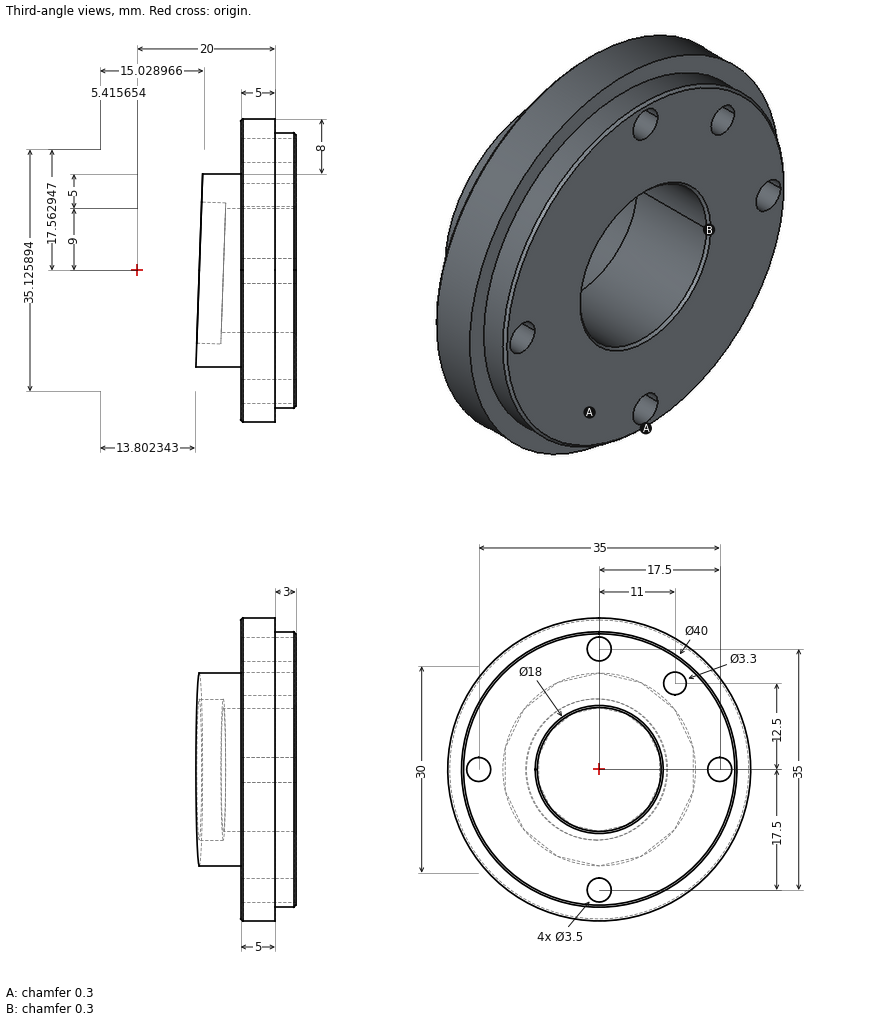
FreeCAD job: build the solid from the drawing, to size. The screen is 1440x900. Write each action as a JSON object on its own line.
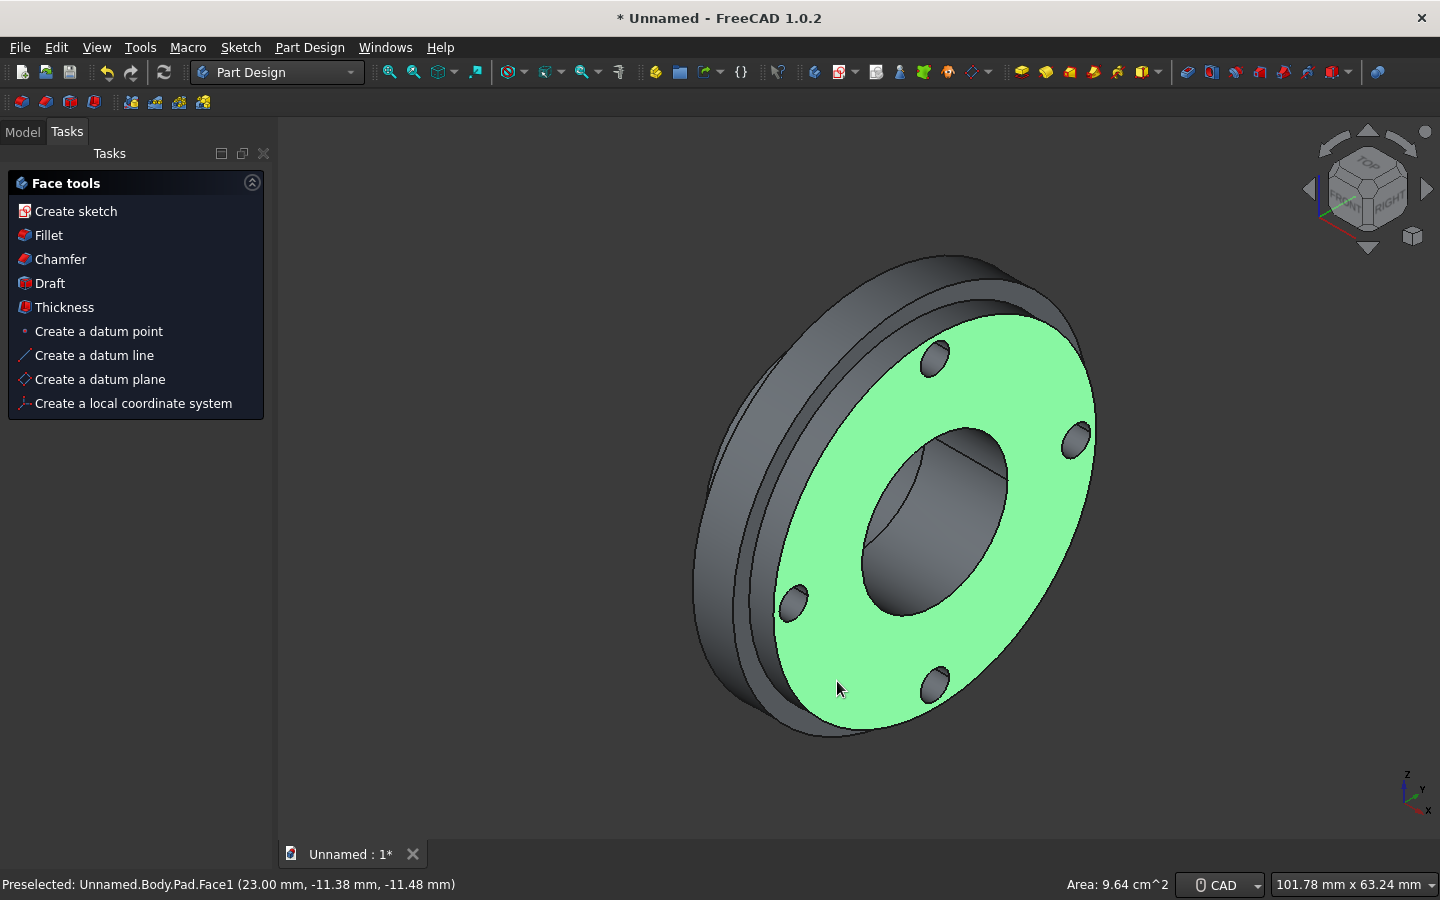
{"action": "left_click", "coordinate": [840, 72]}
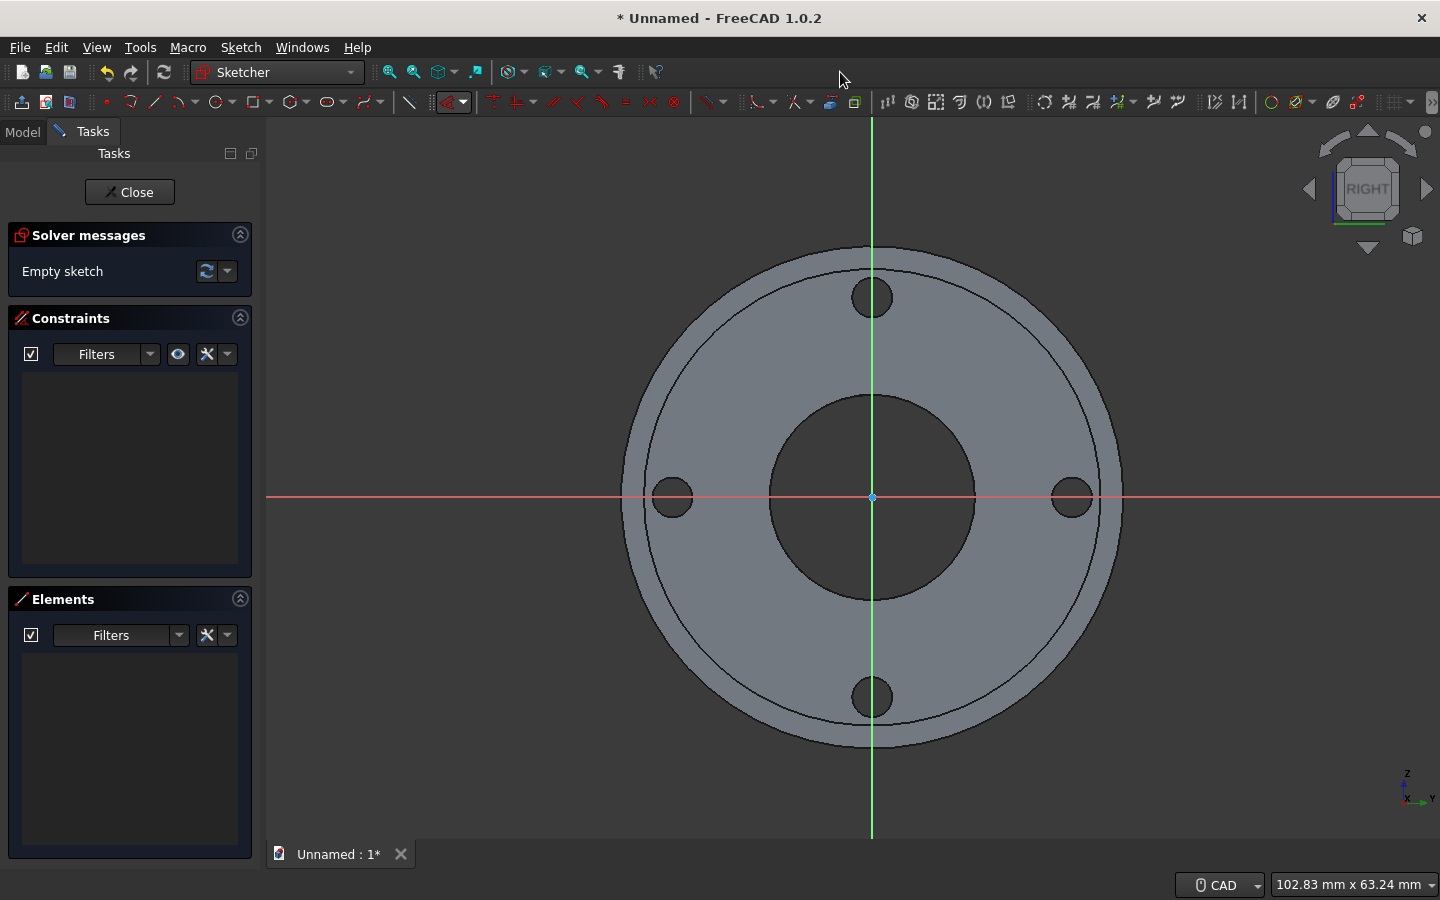
{"action": "scroll", "coordinate": [1015, 345], "scroll_direction": "up", "scroll_amount": 13}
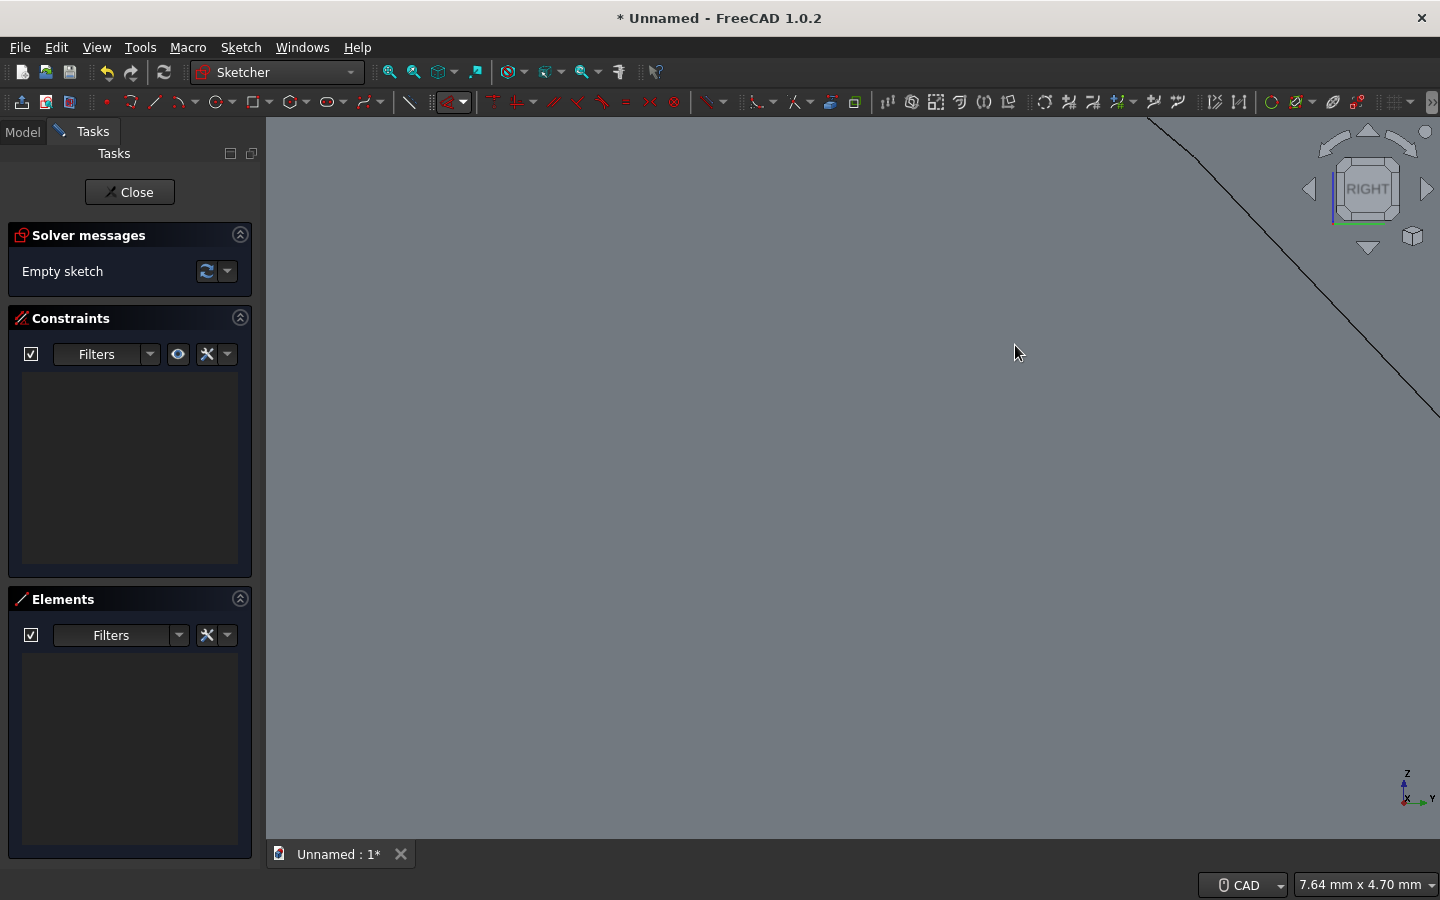
{"action": "key", "text": "g c"}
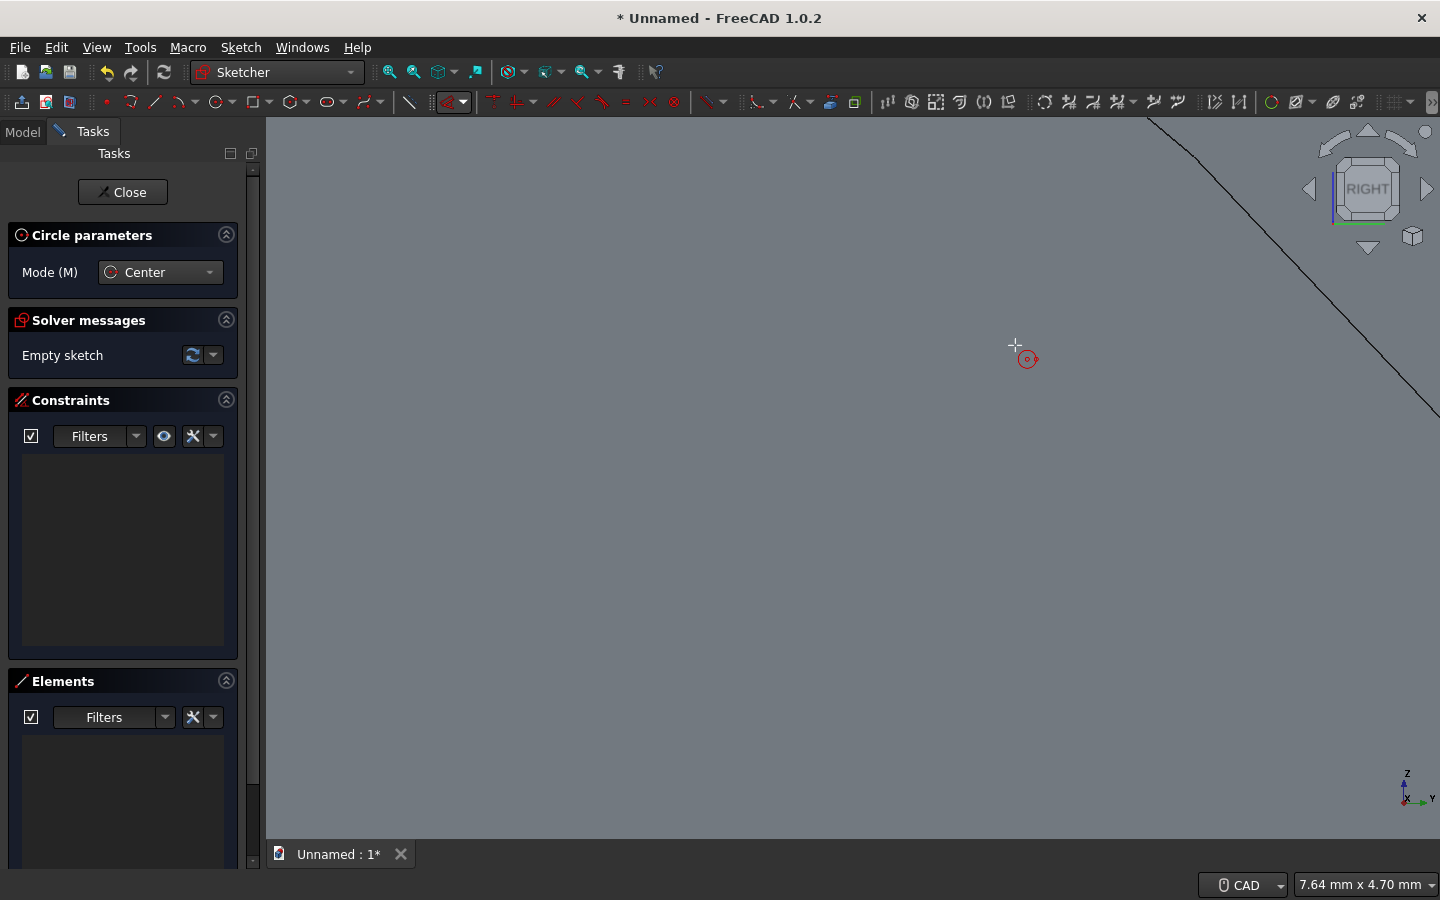
{"action": "left_click", "coordinate": [775, 472]}
{"action": "mouse_move", "coordinate": [955, 292]}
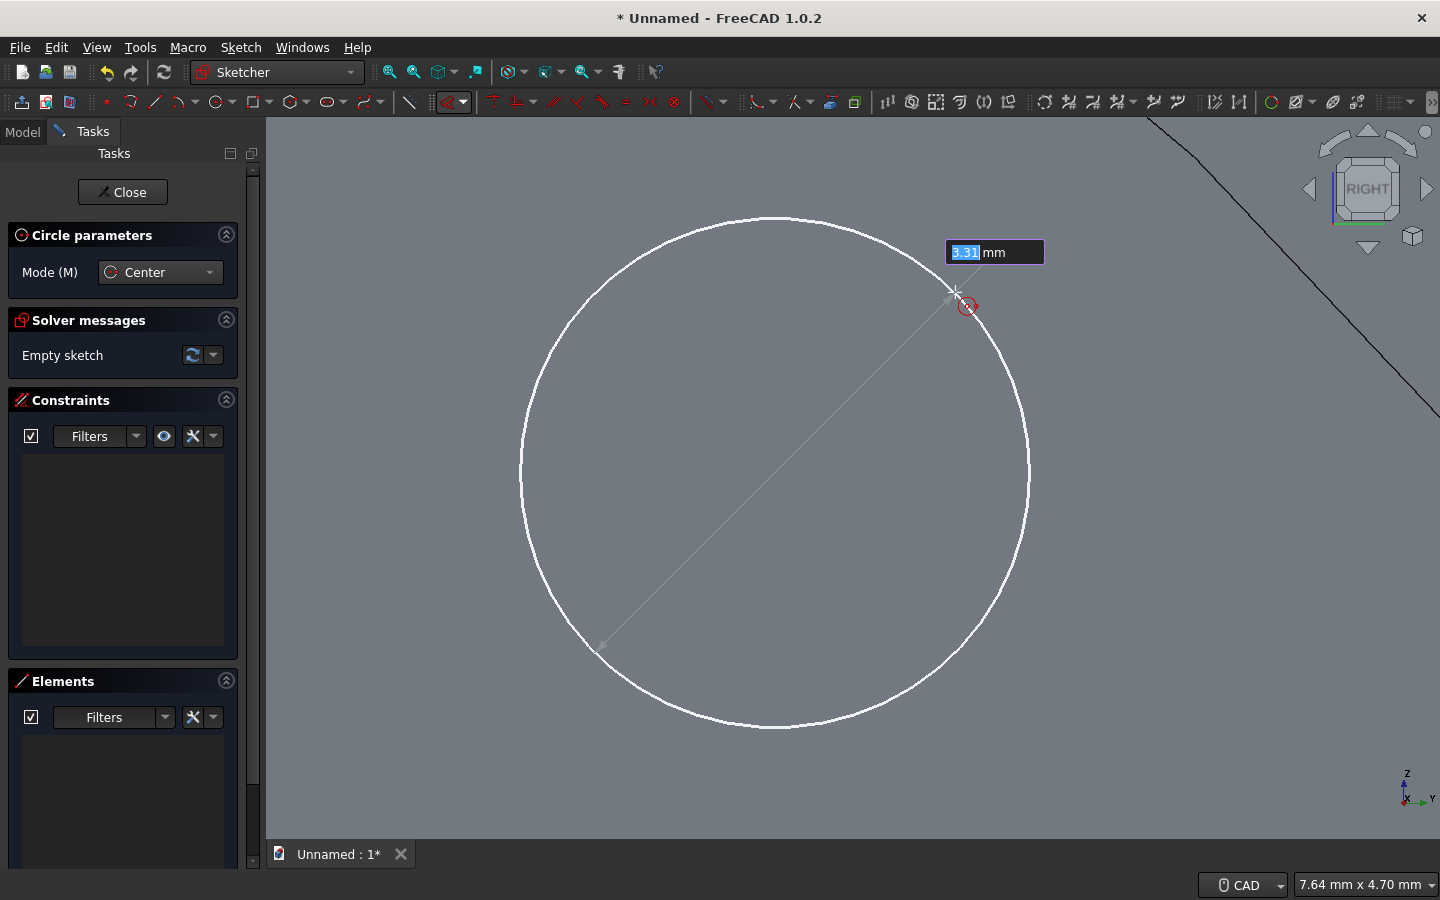
{"action": "type", "text": "3.3"}
{"action": "key", "text": "Return"}
{"action": "key", "text": "Escape"}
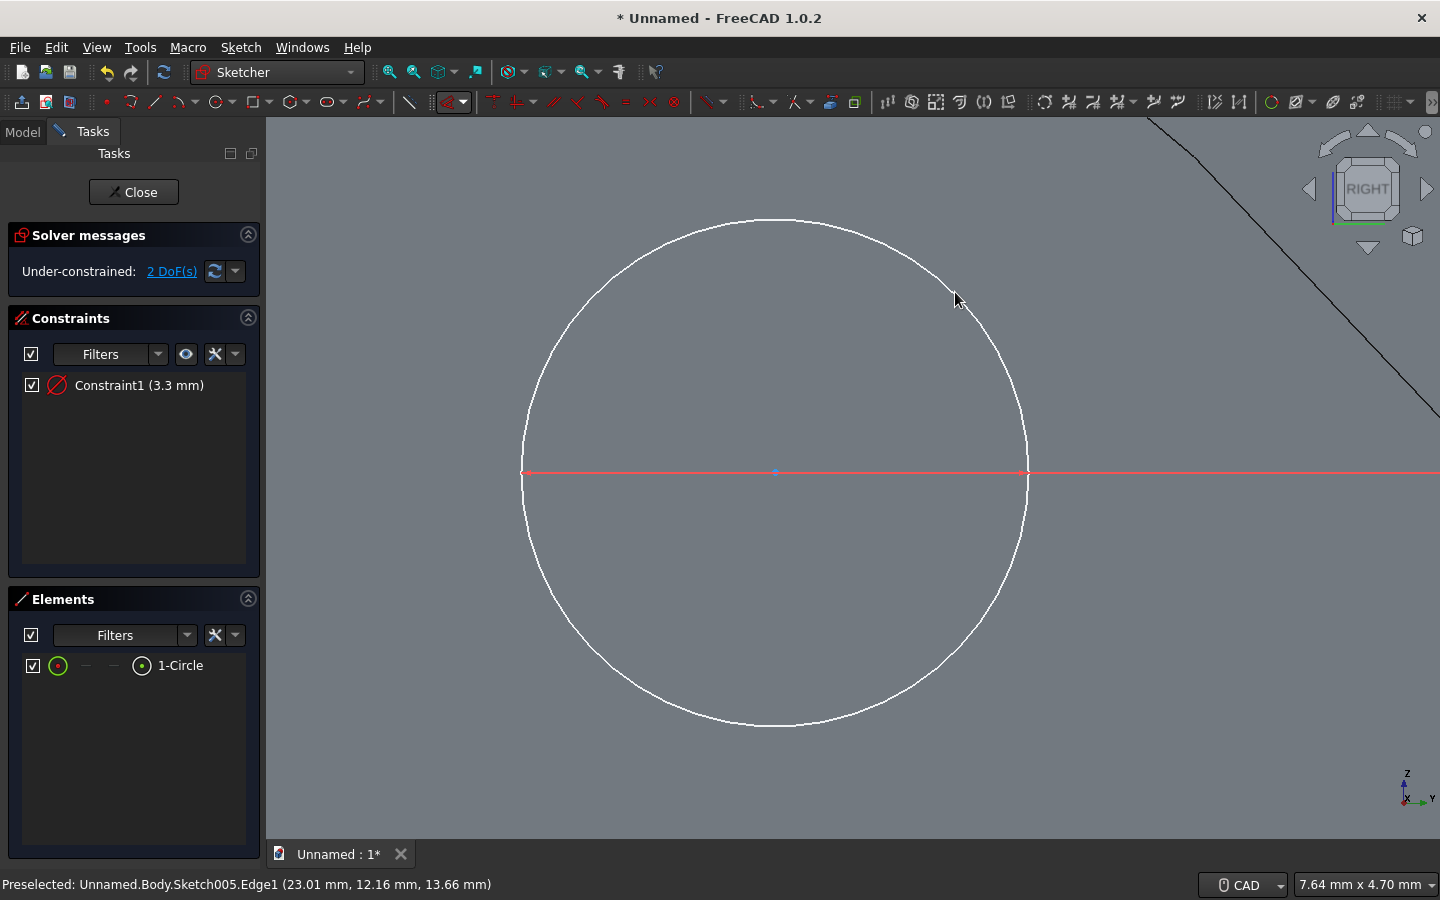
{"action": "left_click", "coordinate": [775, 473]}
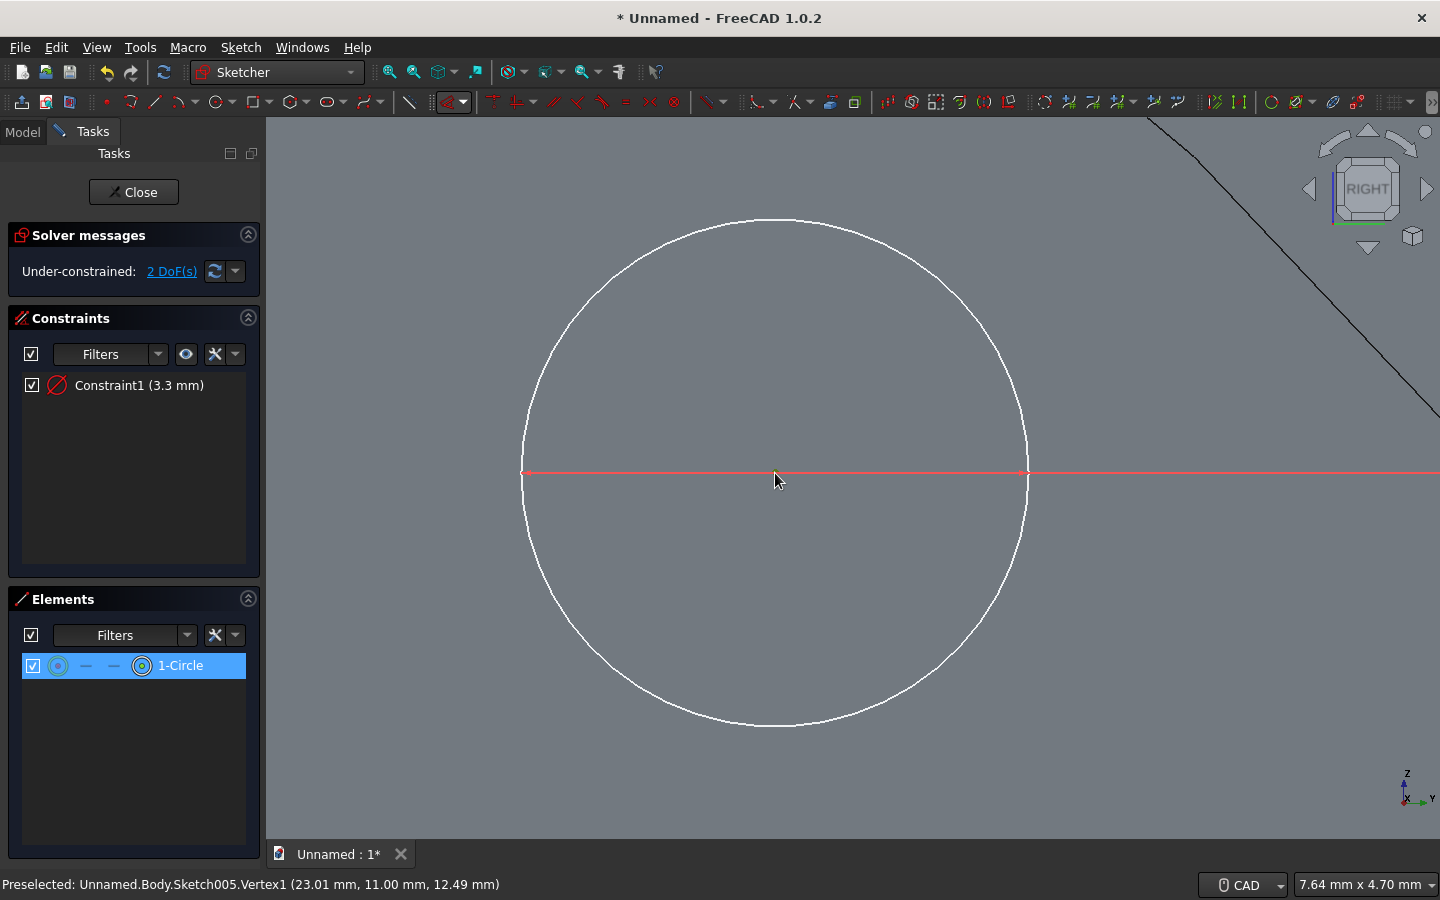
{"action": "left_click", "coordinate": [466, 102]}